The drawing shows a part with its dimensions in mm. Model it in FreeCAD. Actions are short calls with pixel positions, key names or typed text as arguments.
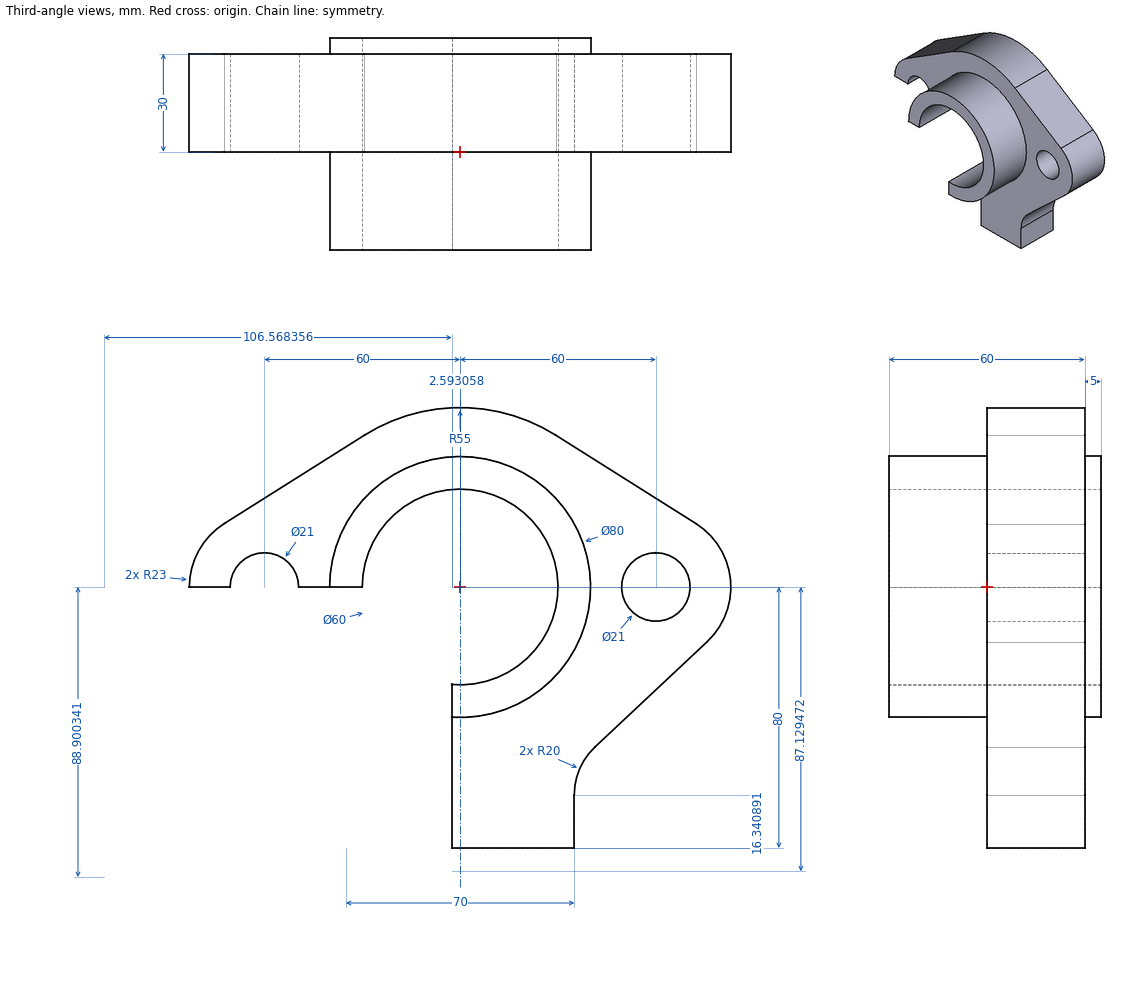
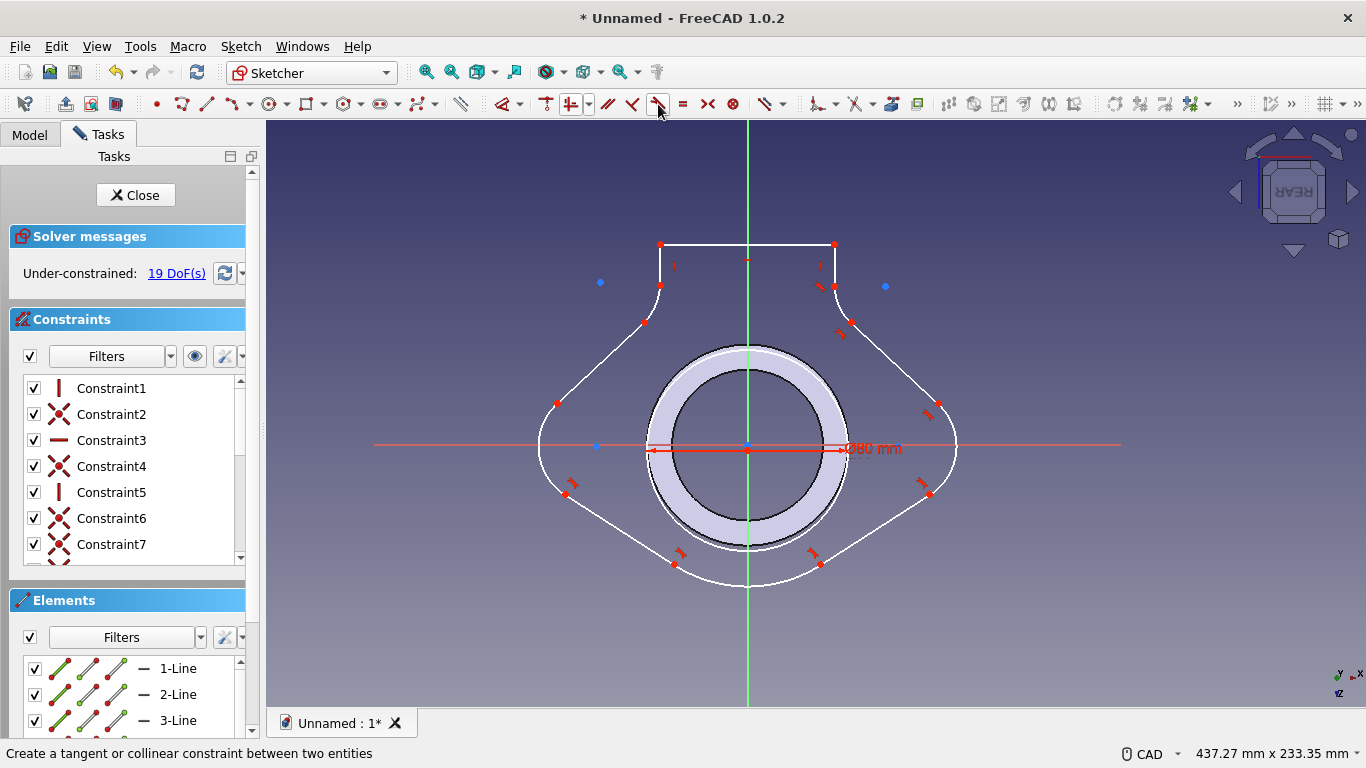
click(660, 257)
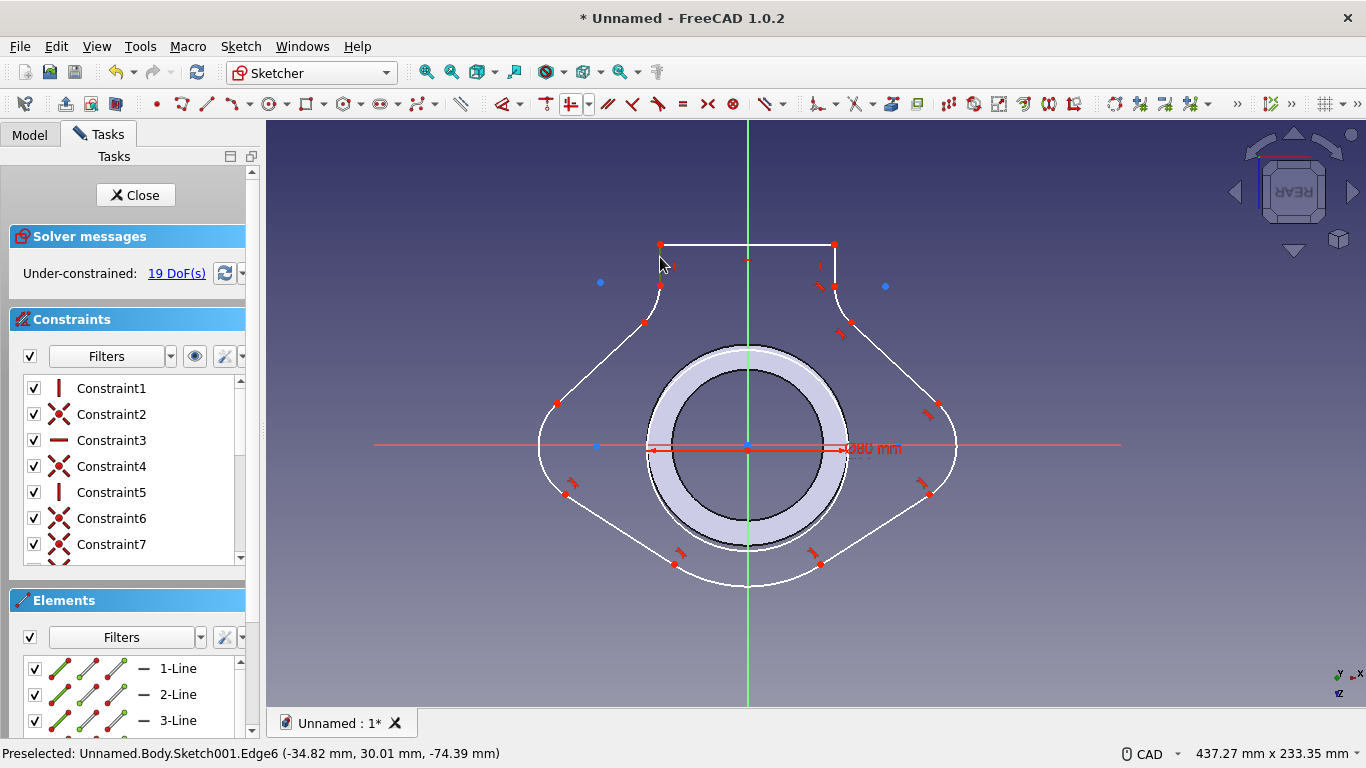
click(651, 313)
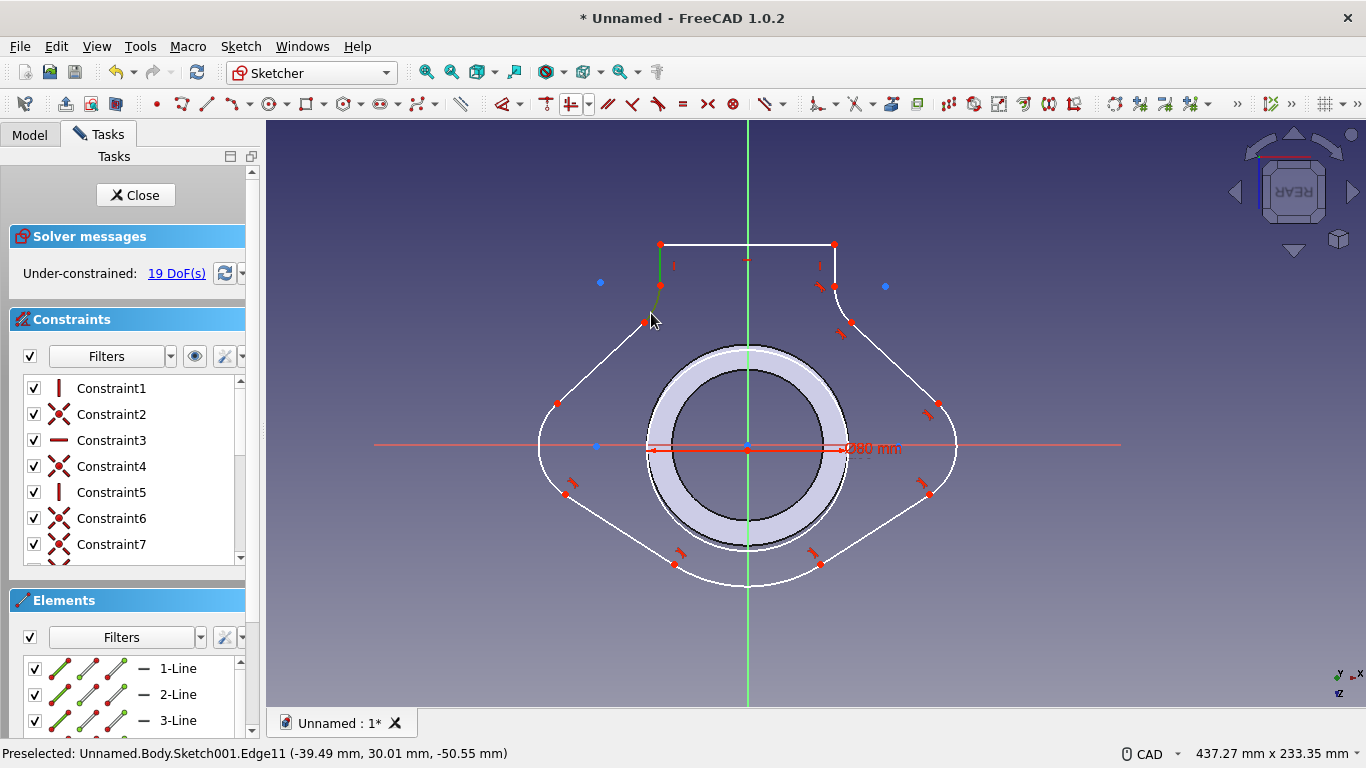
click(658, 104)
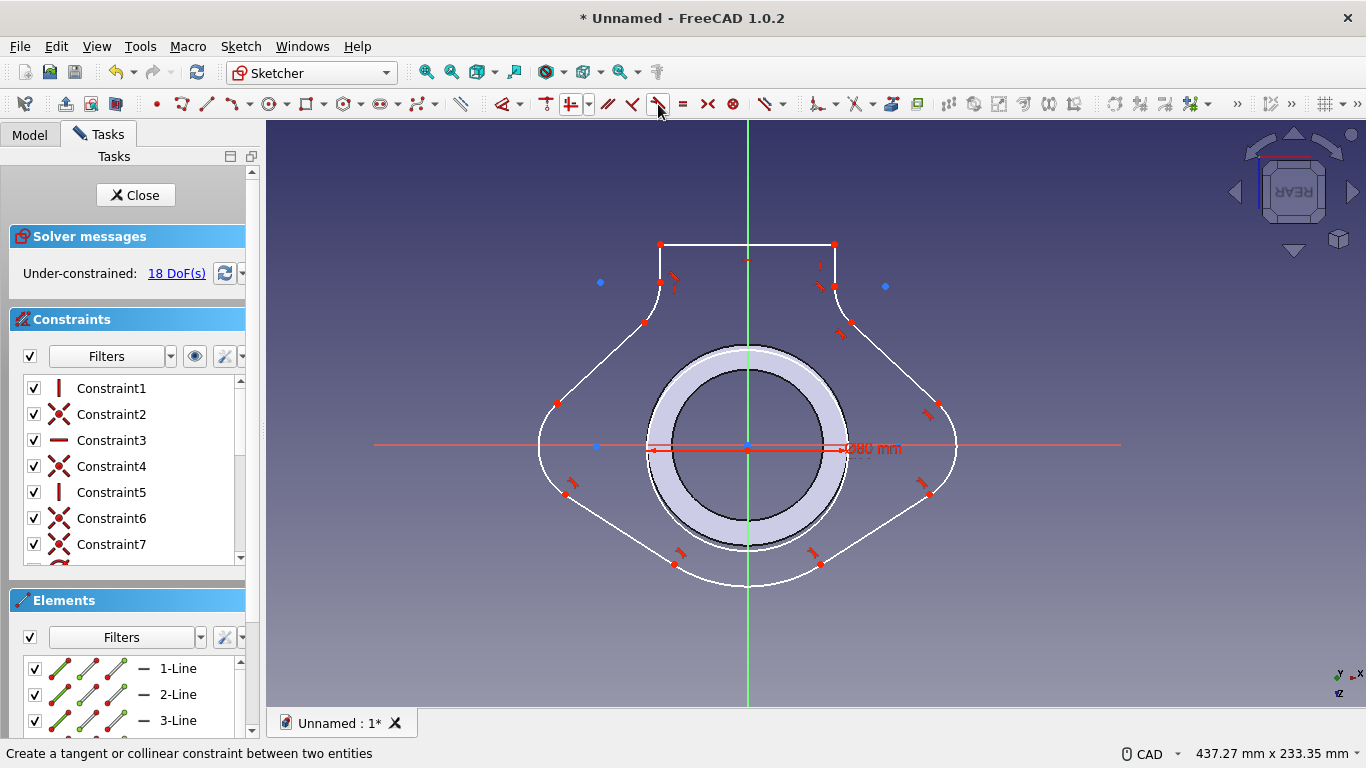
click(618, 347)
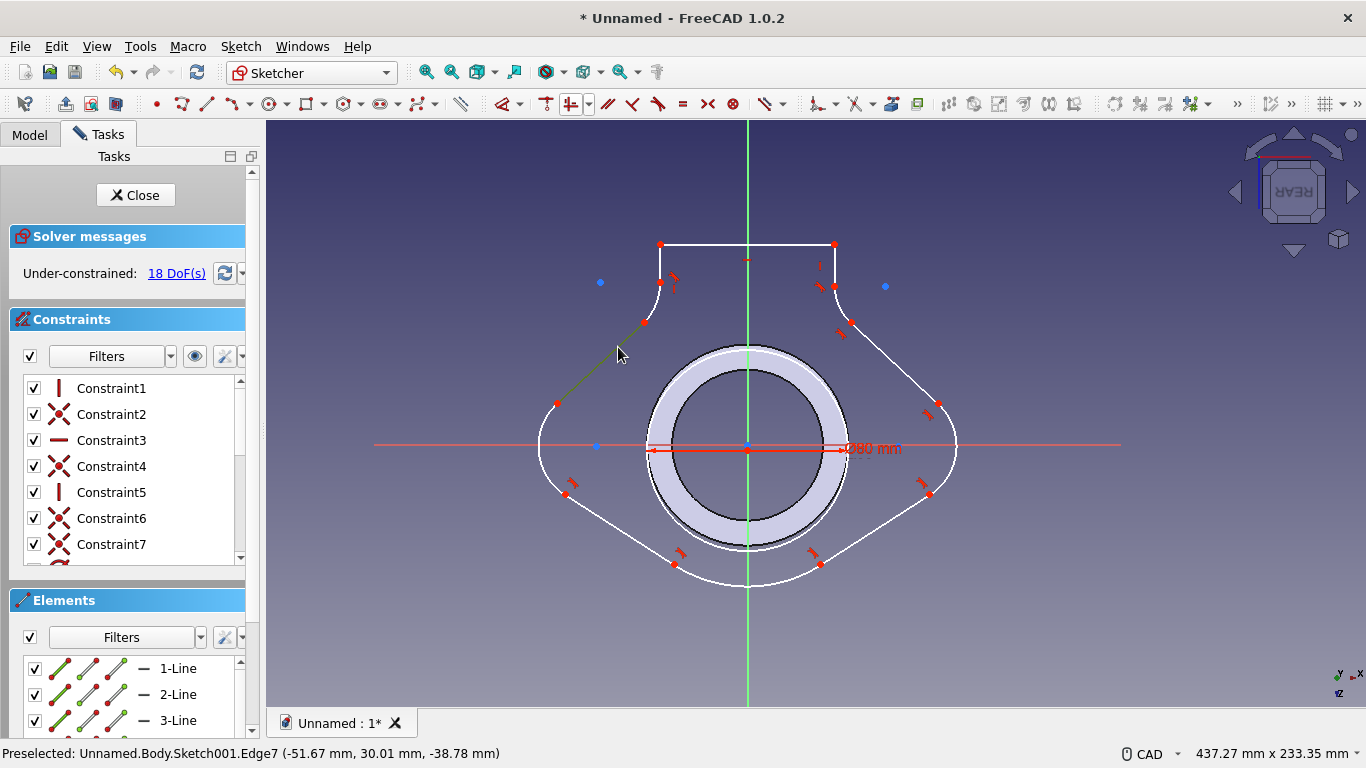
click(652, 312)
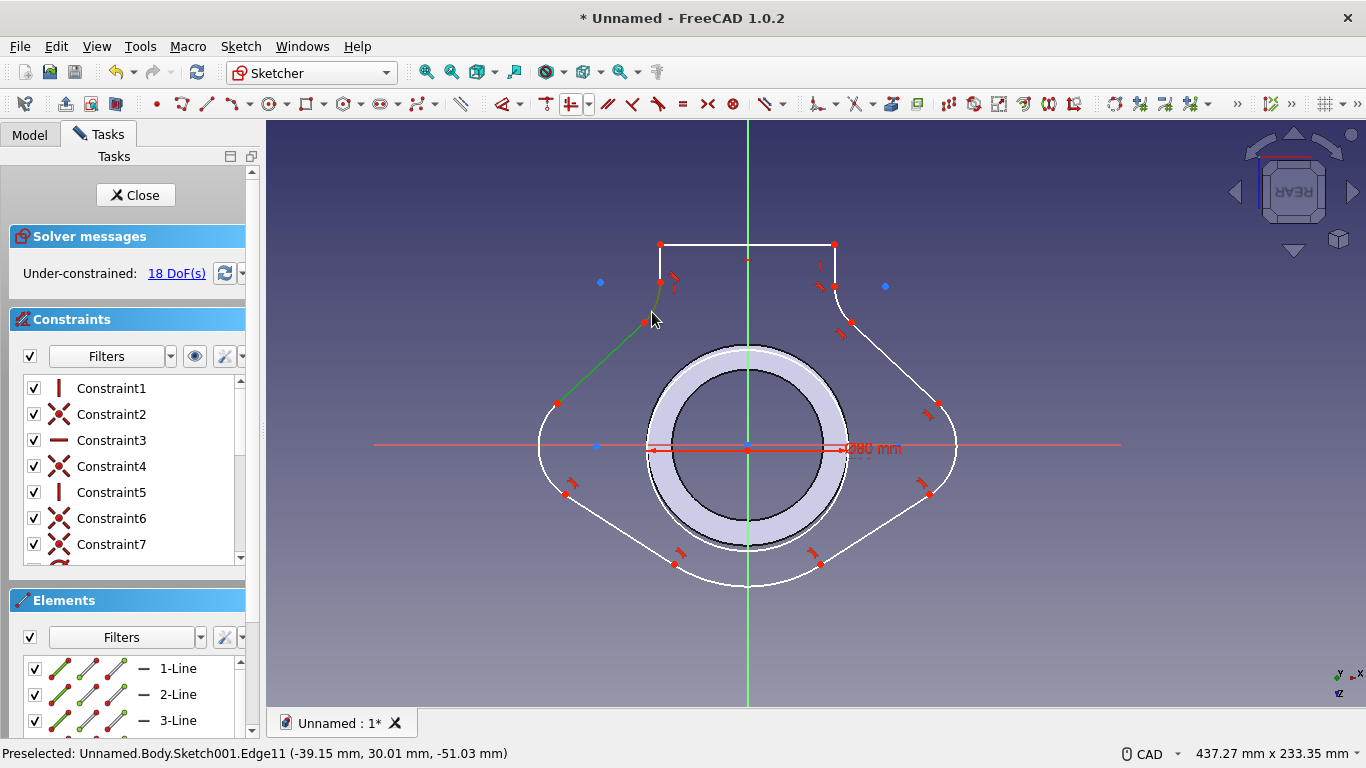
click(658, 104)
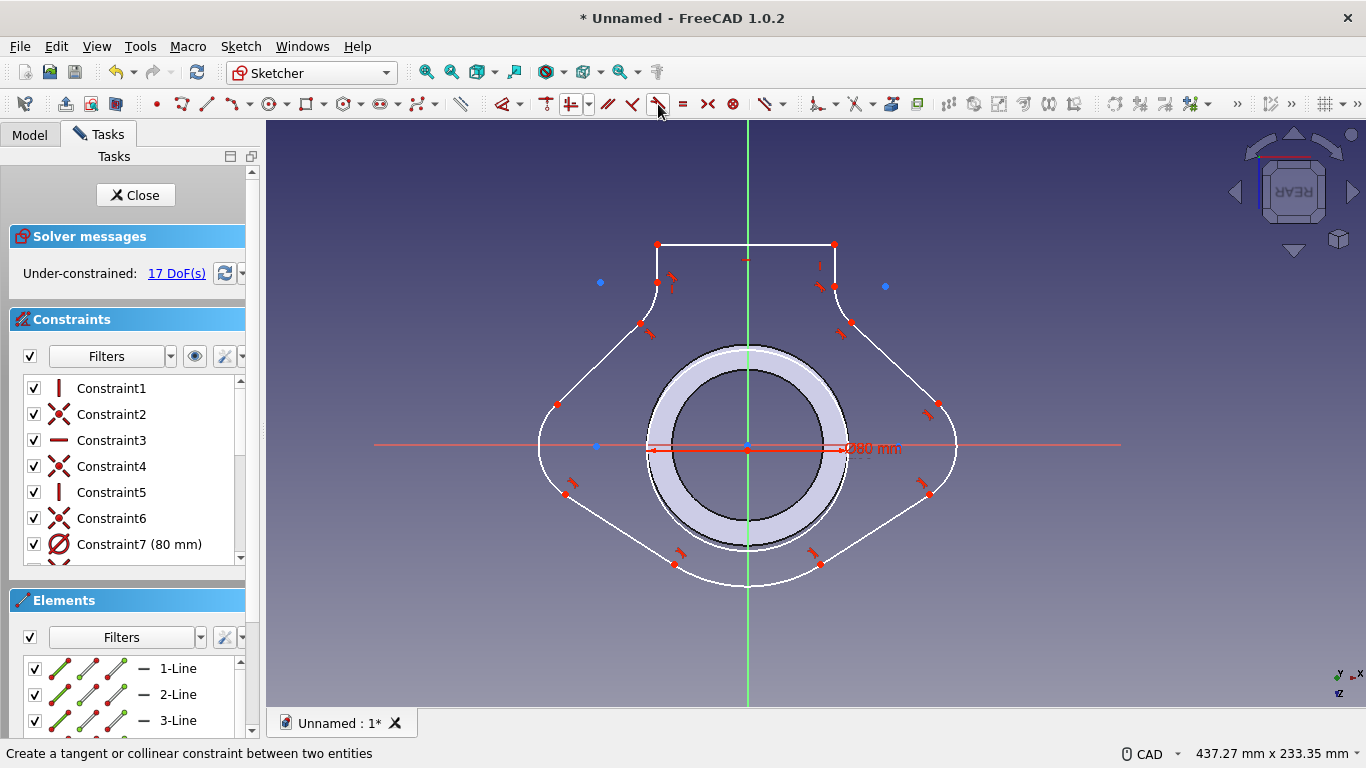
click(615, 347)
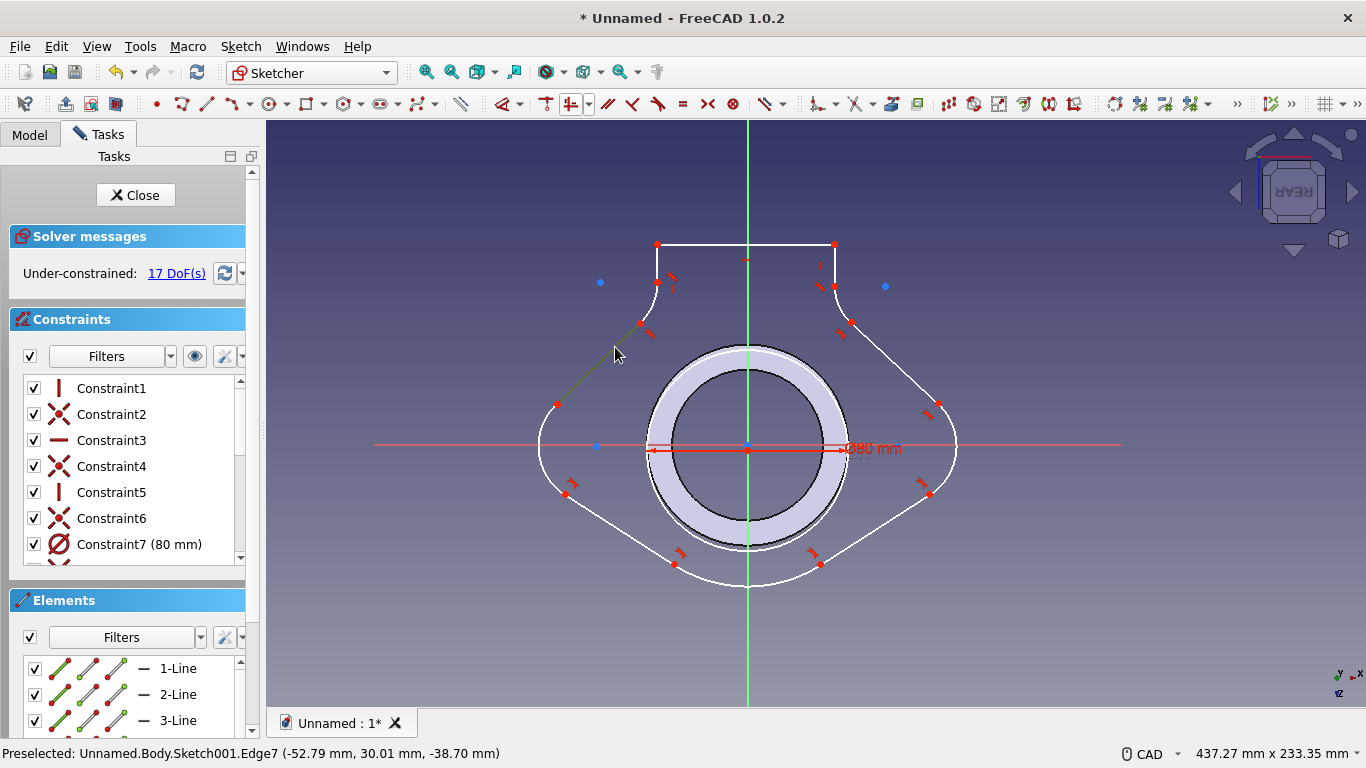
click(541, 431)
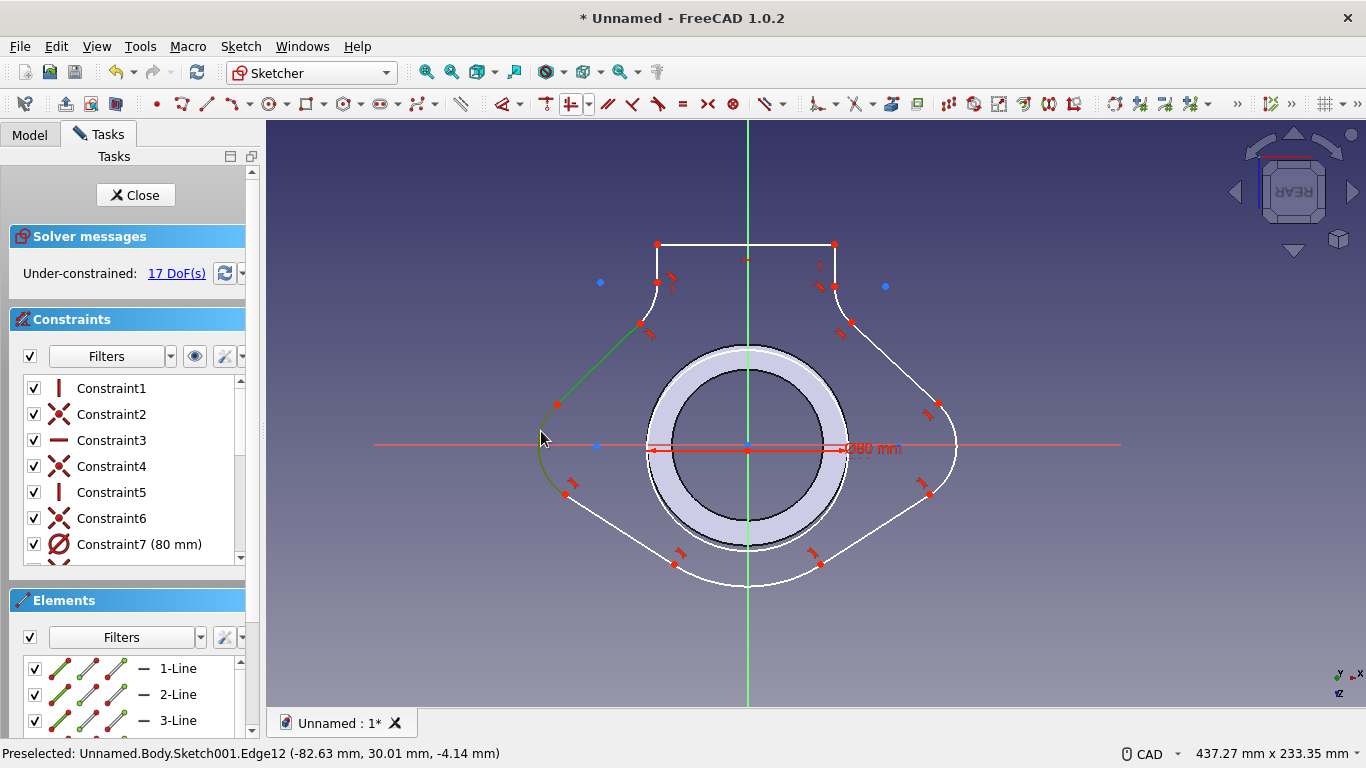
click(658, 104)